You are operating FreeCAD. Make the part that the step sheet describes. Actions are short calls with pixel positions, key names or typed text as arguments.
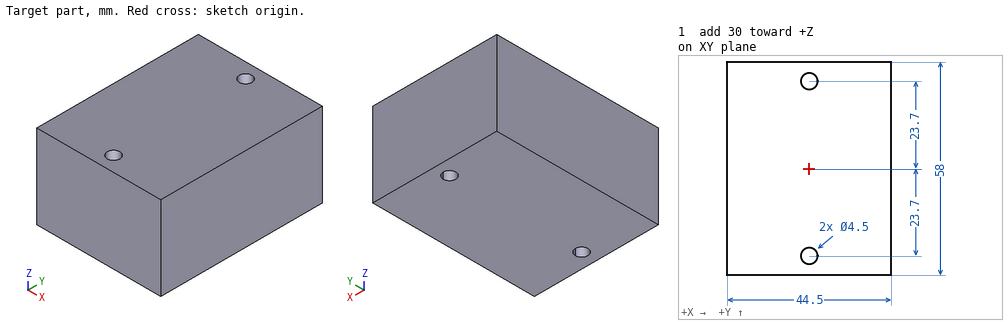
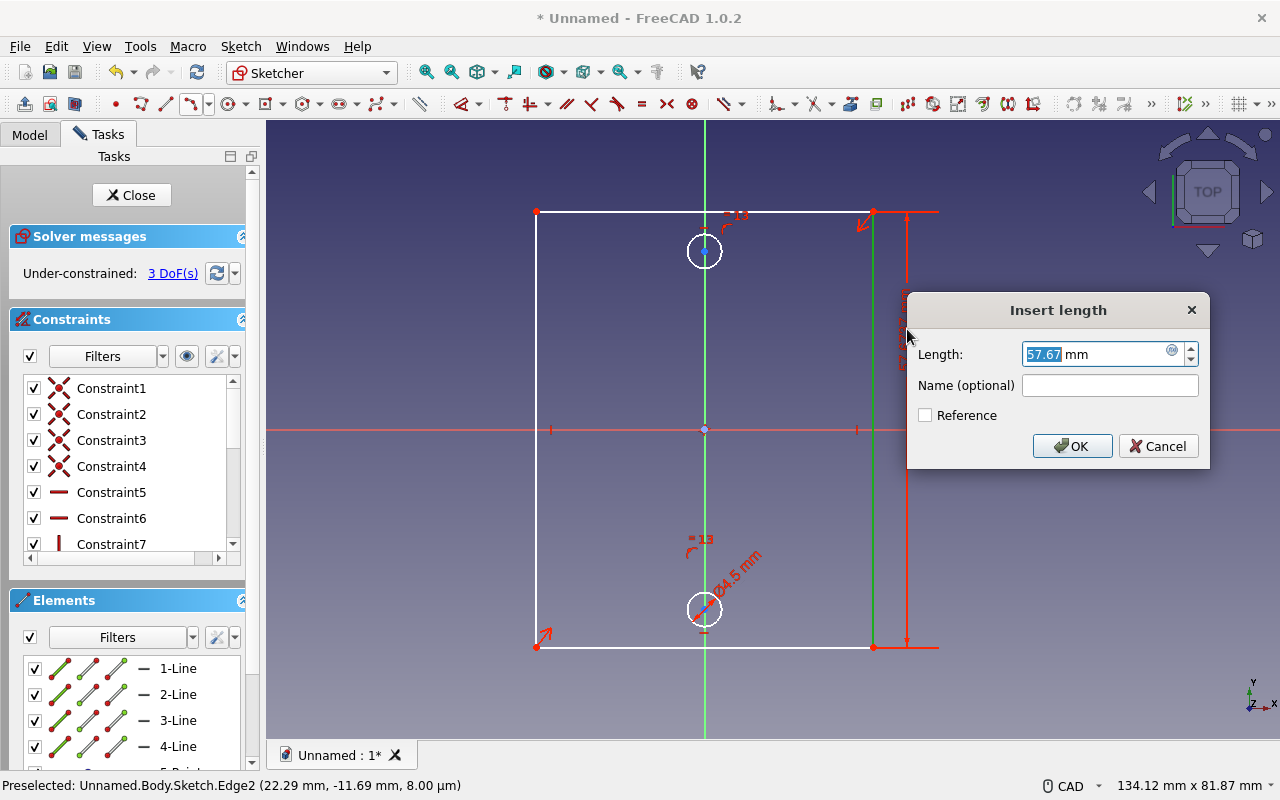
text(58)
key(Return)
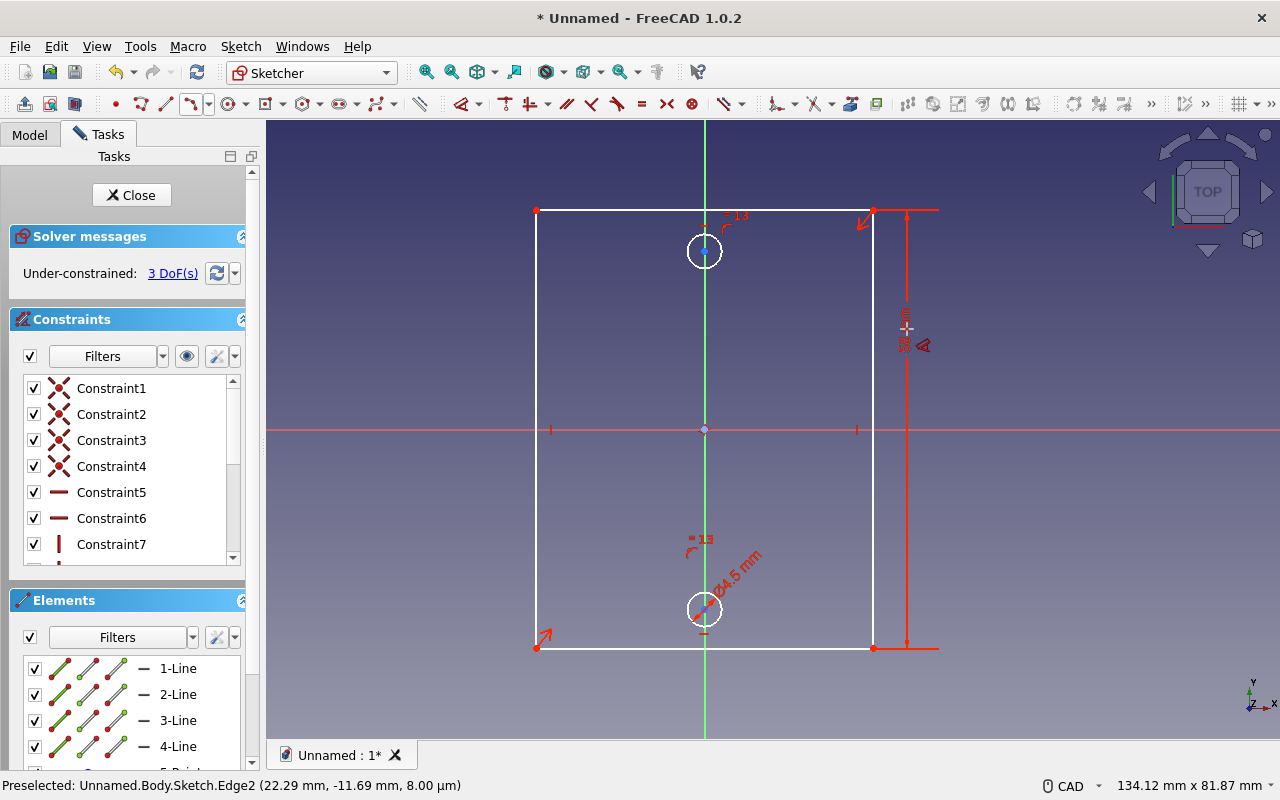
click(637, 649)
click(627, 683)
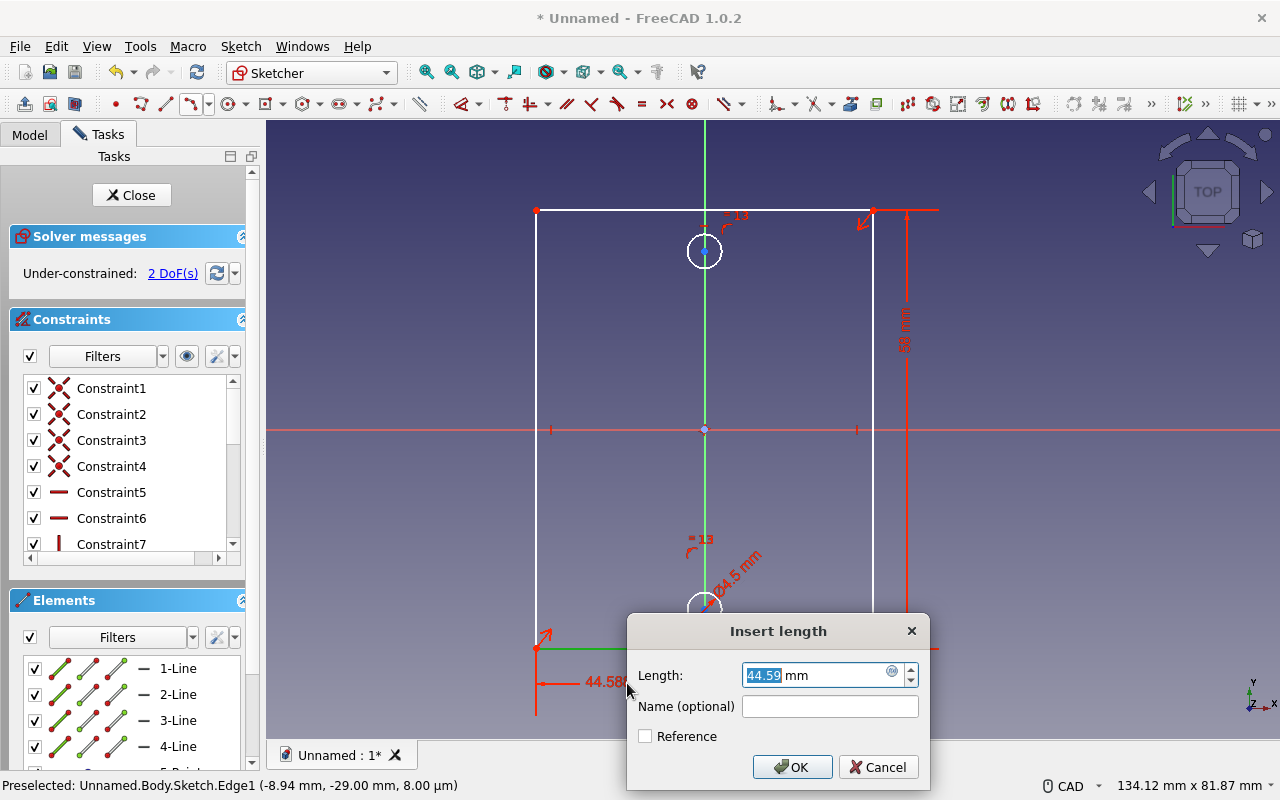
text(44.5)
key(Return)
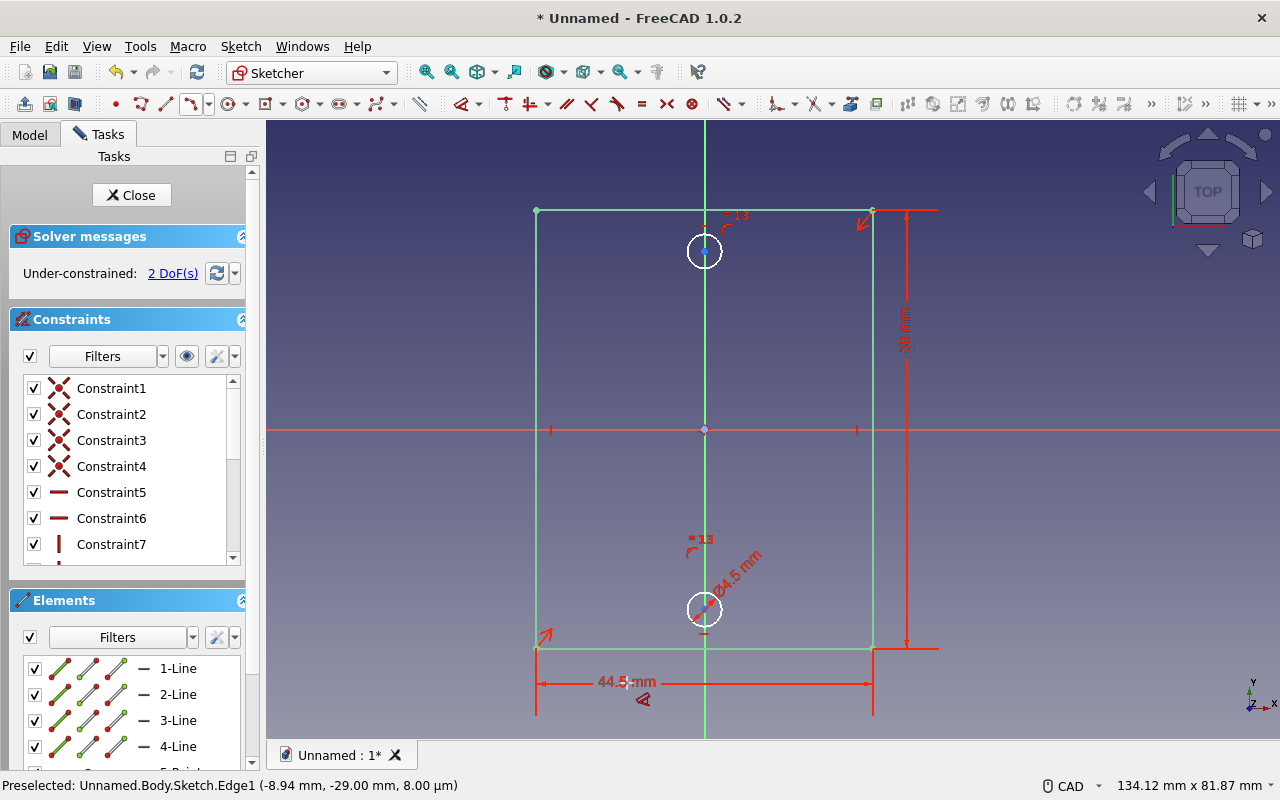
click(705, 610)
click(739, 520)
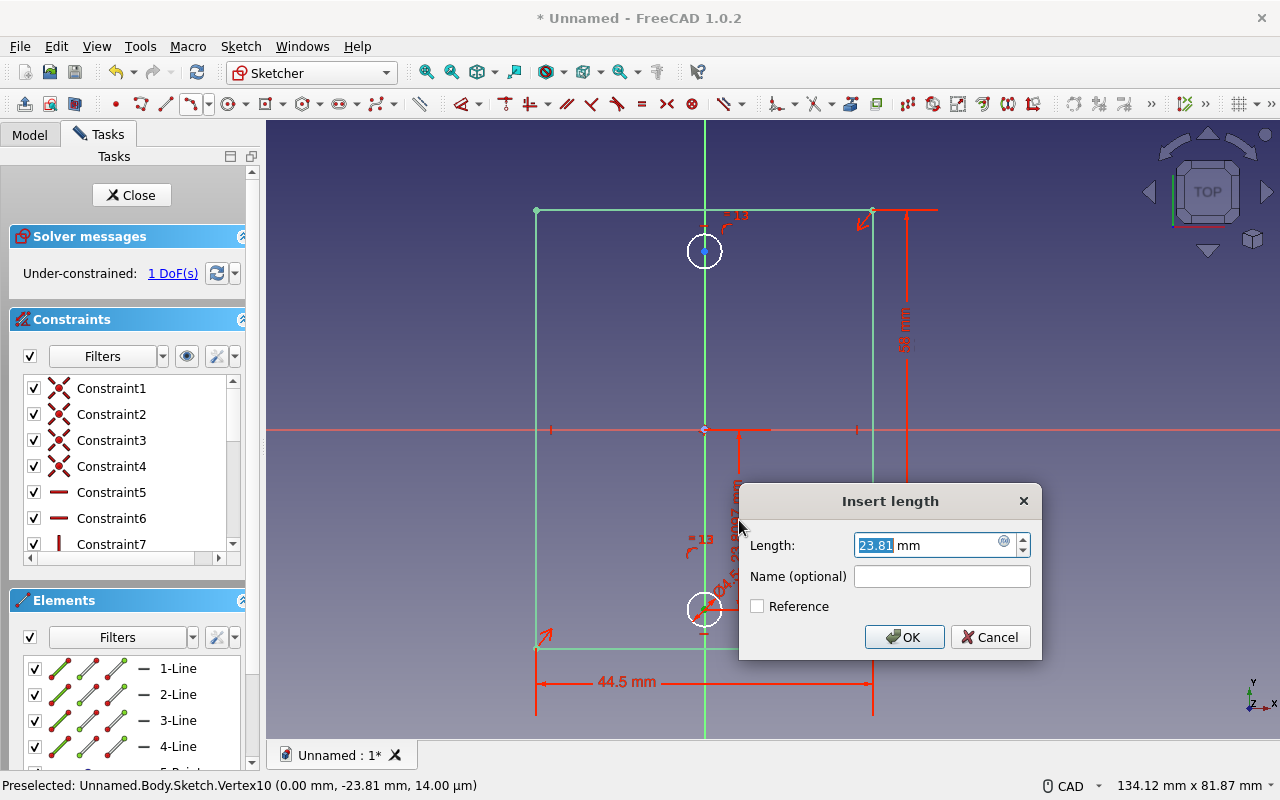
text(23.7)
key(Return)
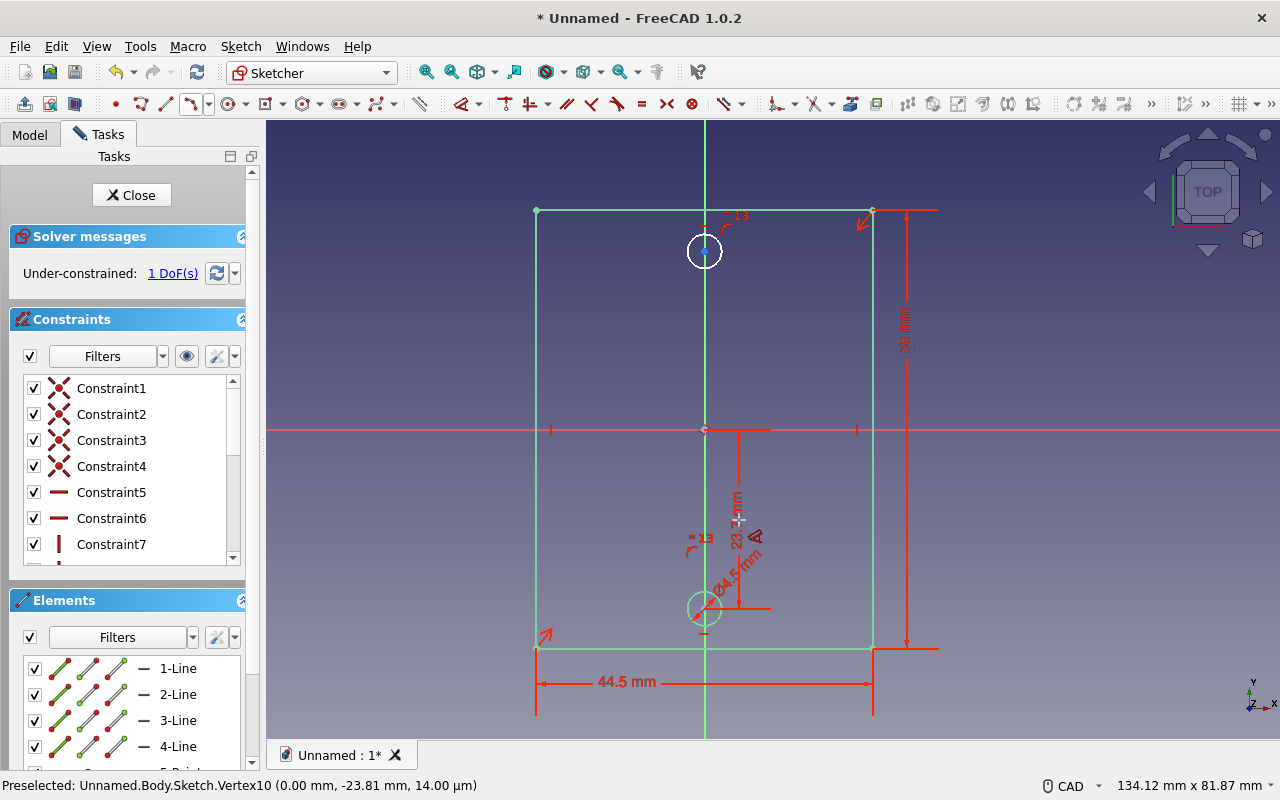
click(705, 251)
click(739, 341)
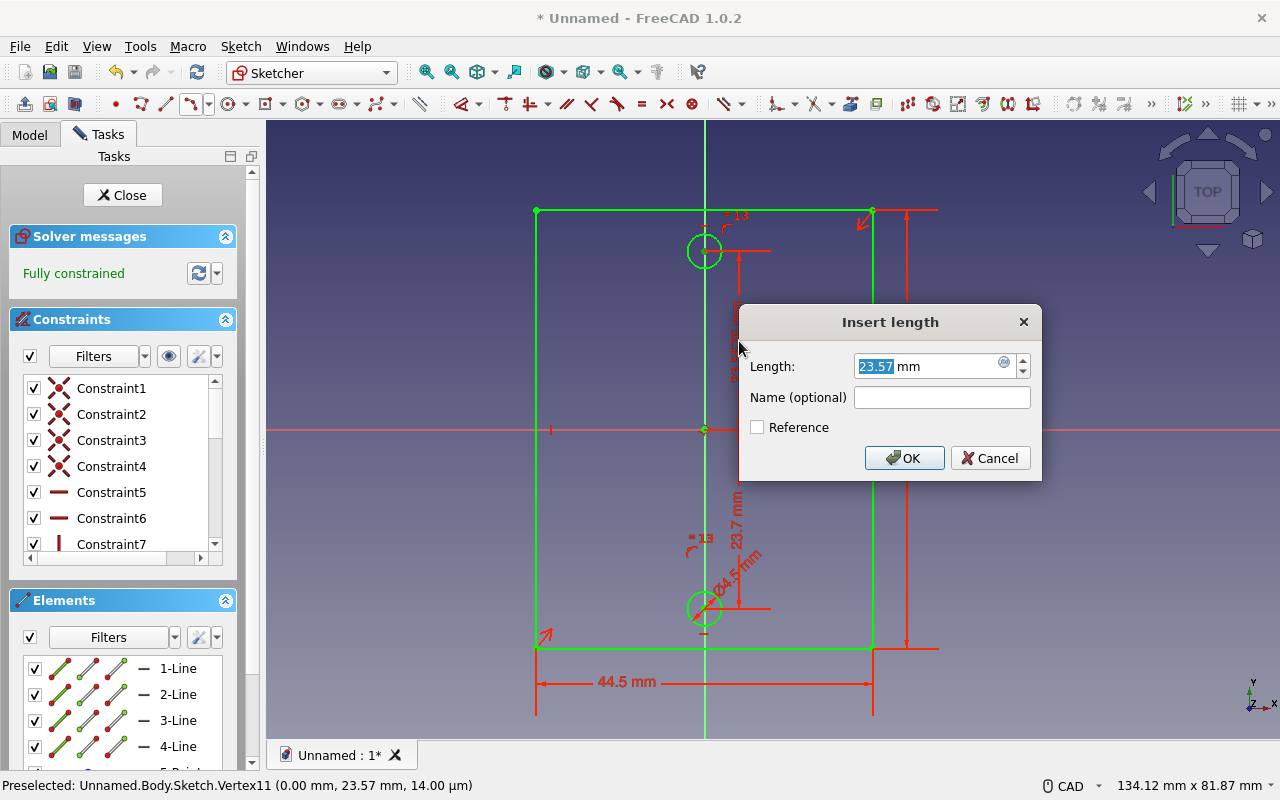
text(23.7)
key(Return)
key(Escape)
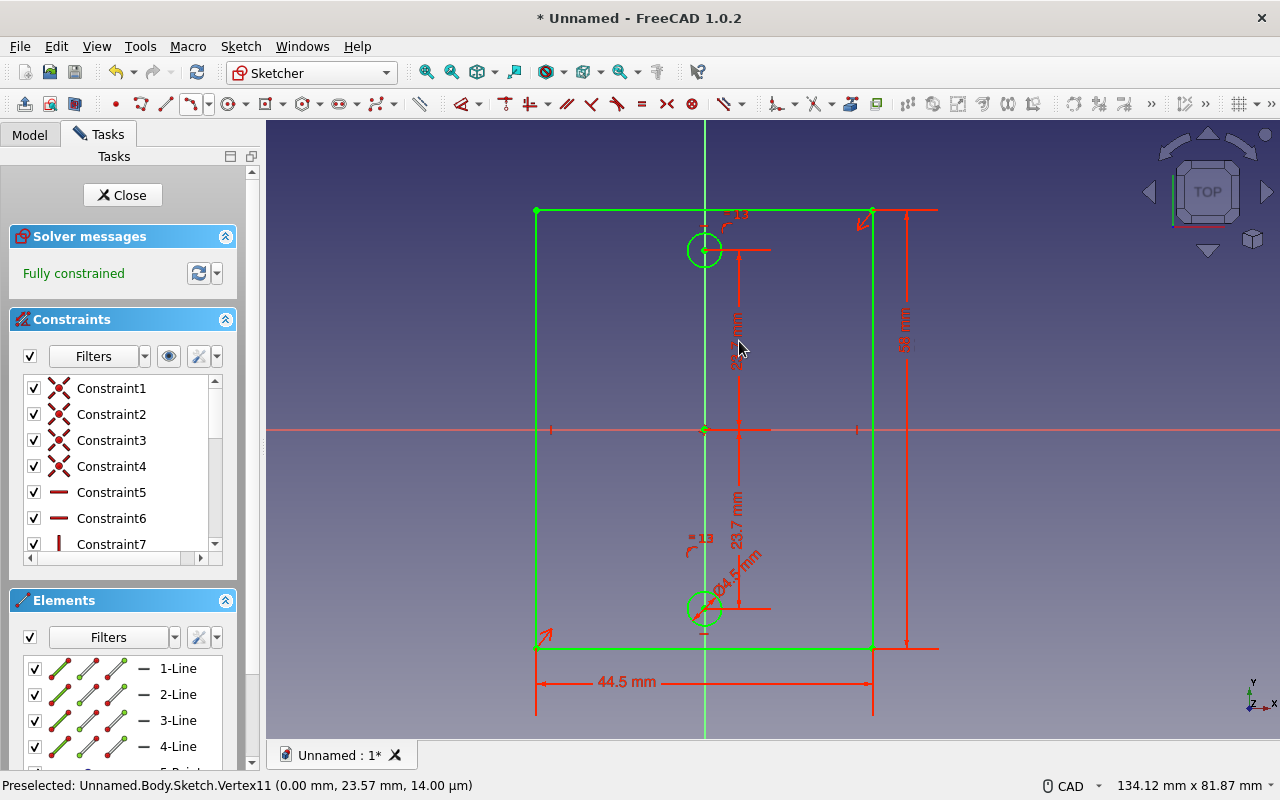
click(123, 195)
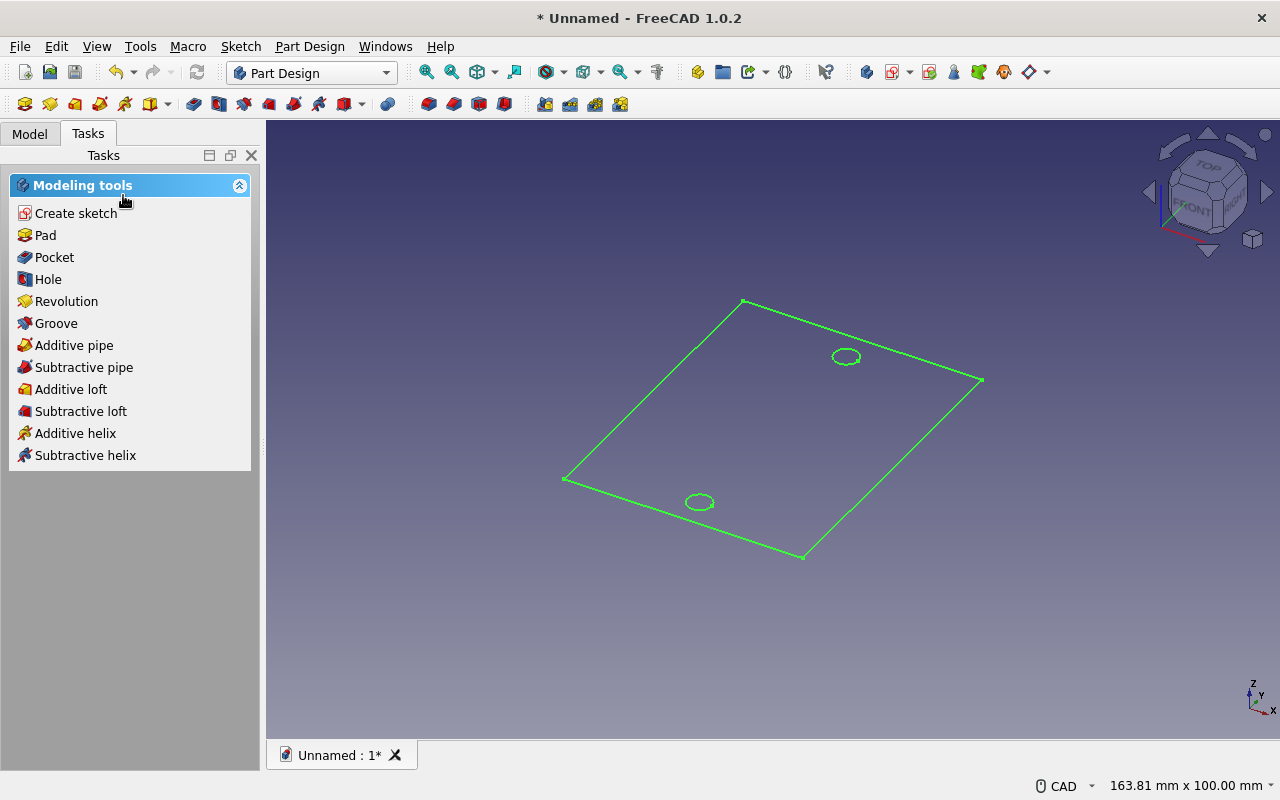
click(25, 104)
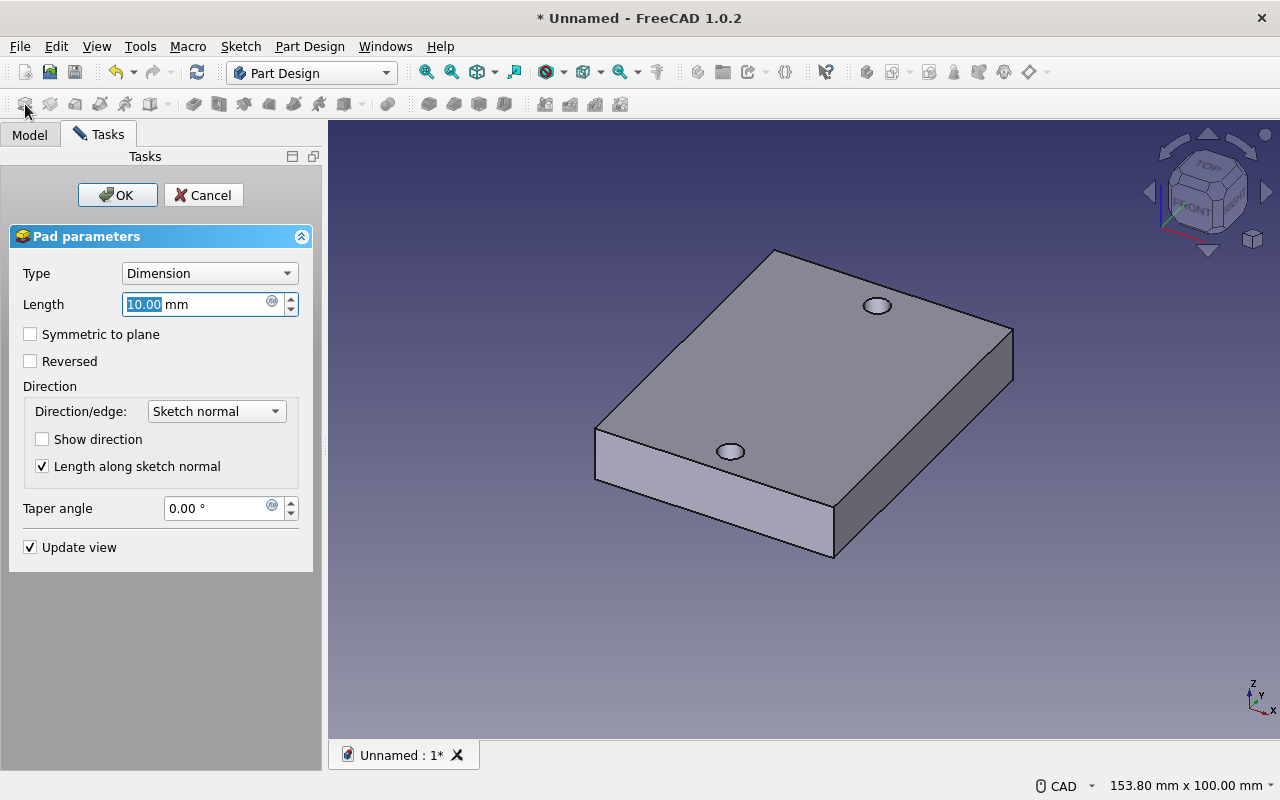
text(30)
key(Tab)